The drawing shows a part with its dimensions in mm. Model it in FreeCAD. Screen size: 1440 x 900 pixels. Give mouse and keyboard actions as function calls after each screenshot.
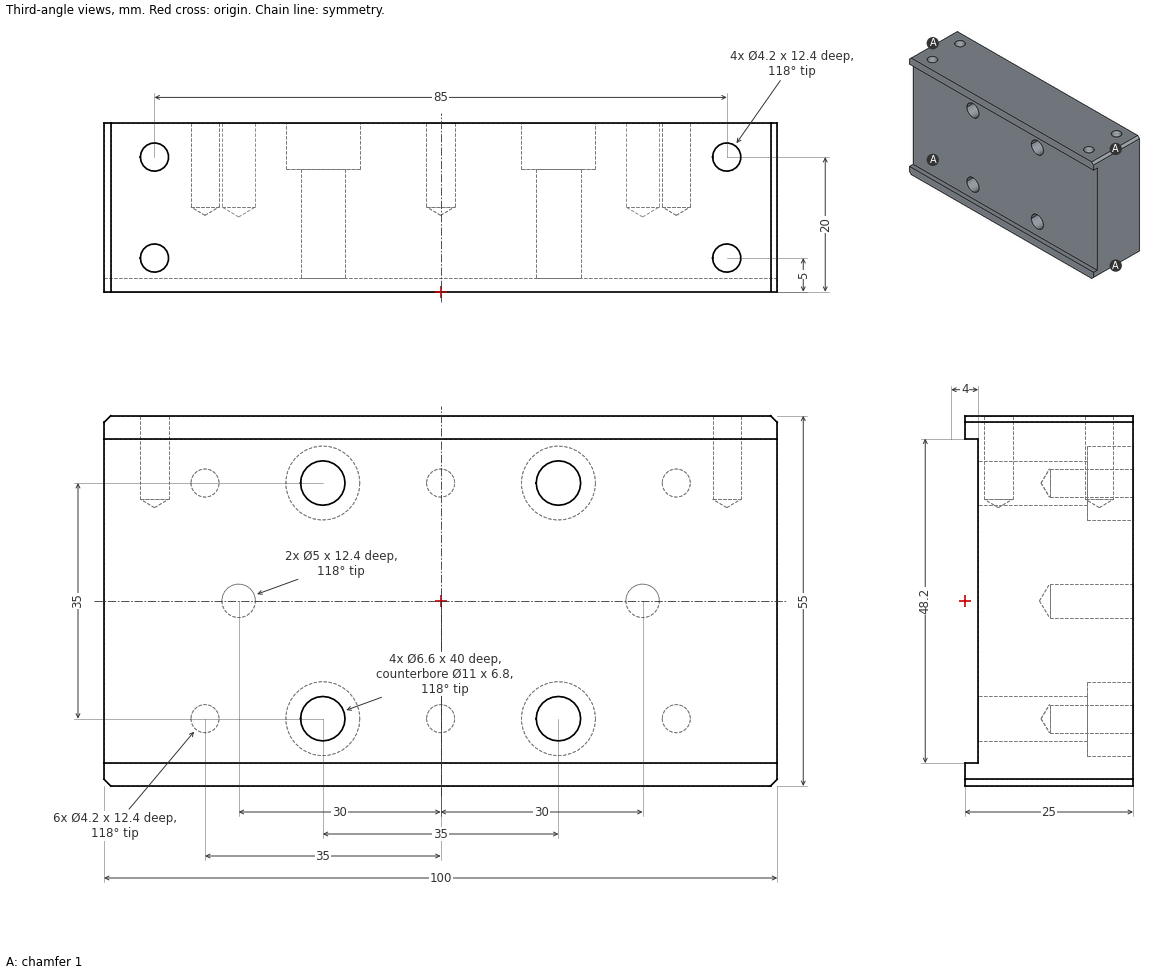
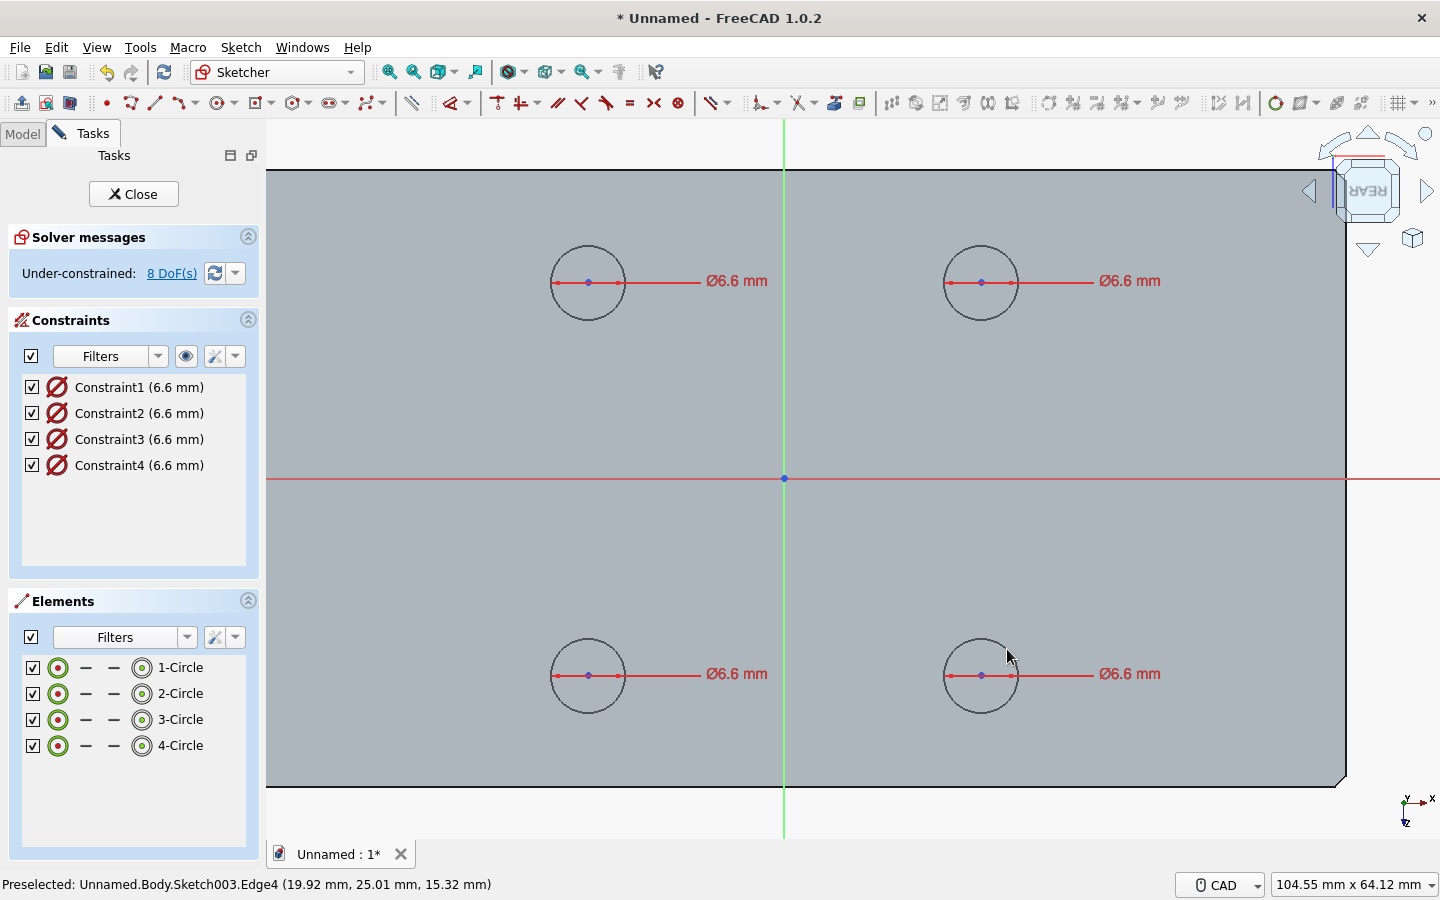
click(588, 283)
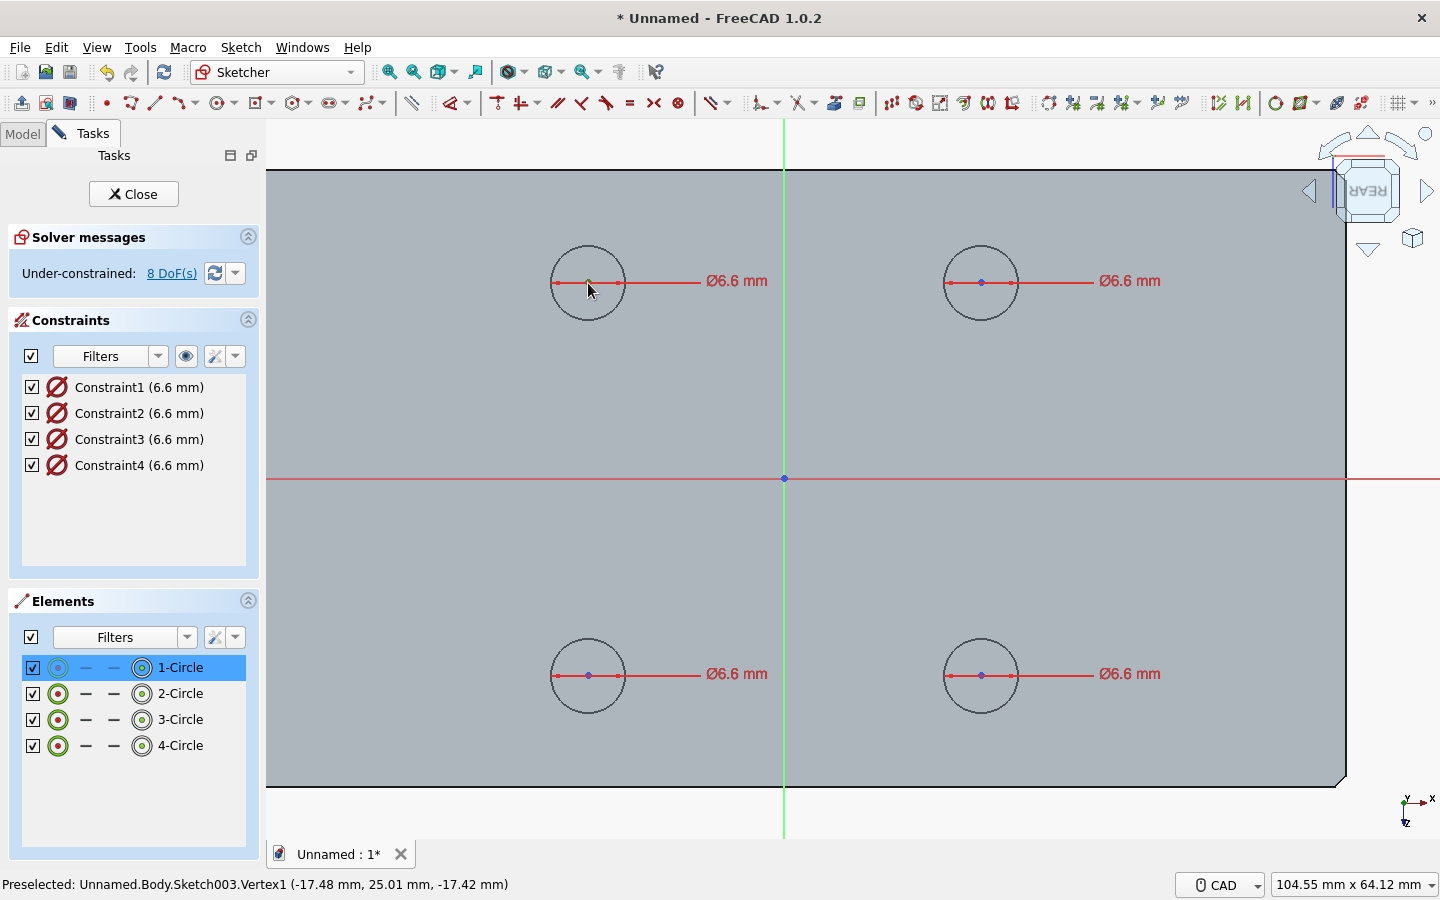
click(981, 283)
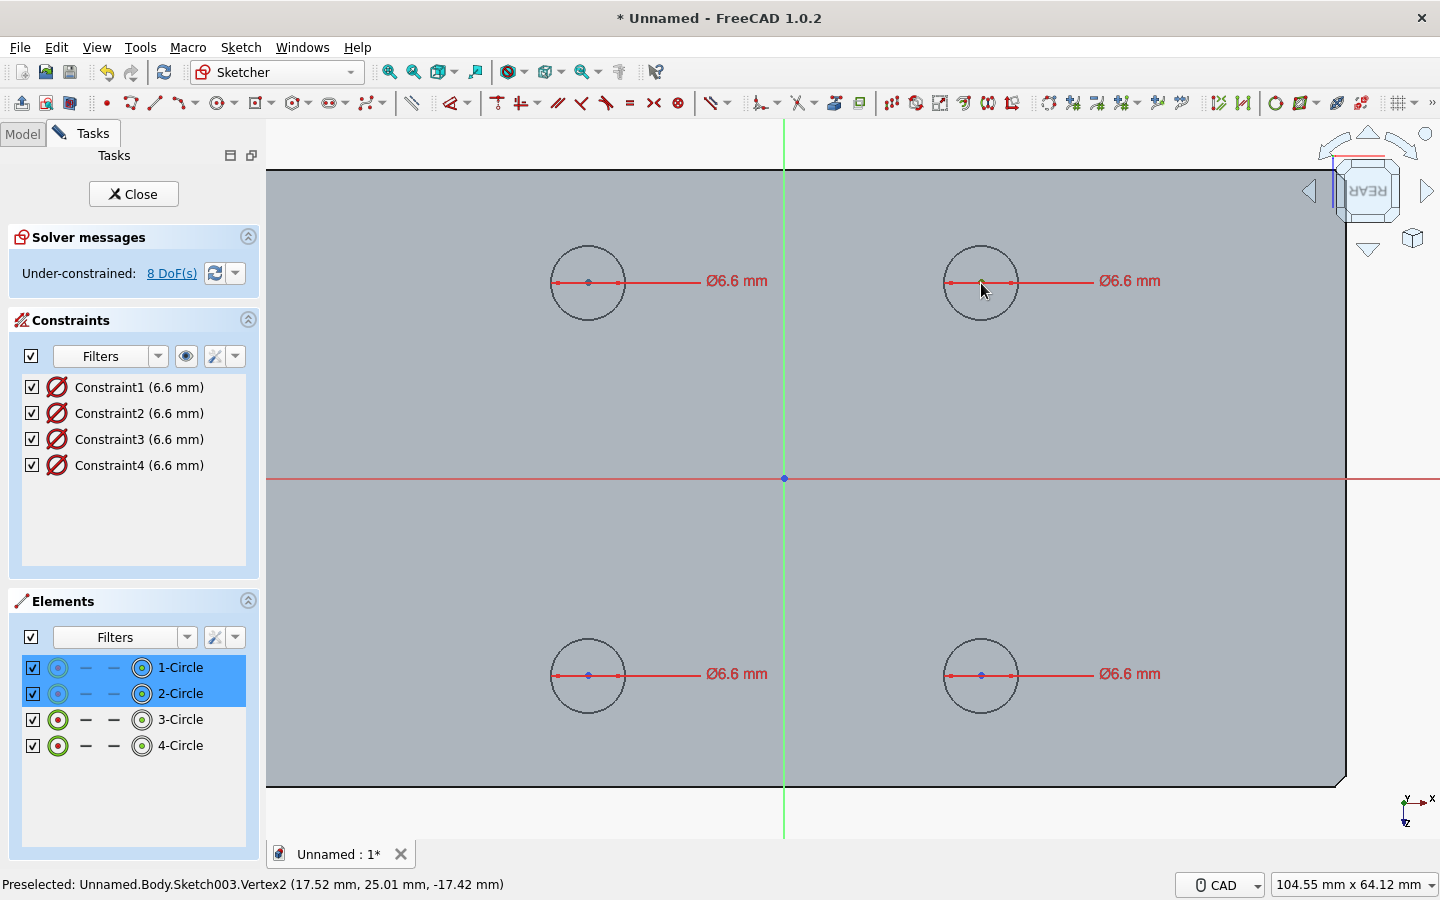
click(784, 764)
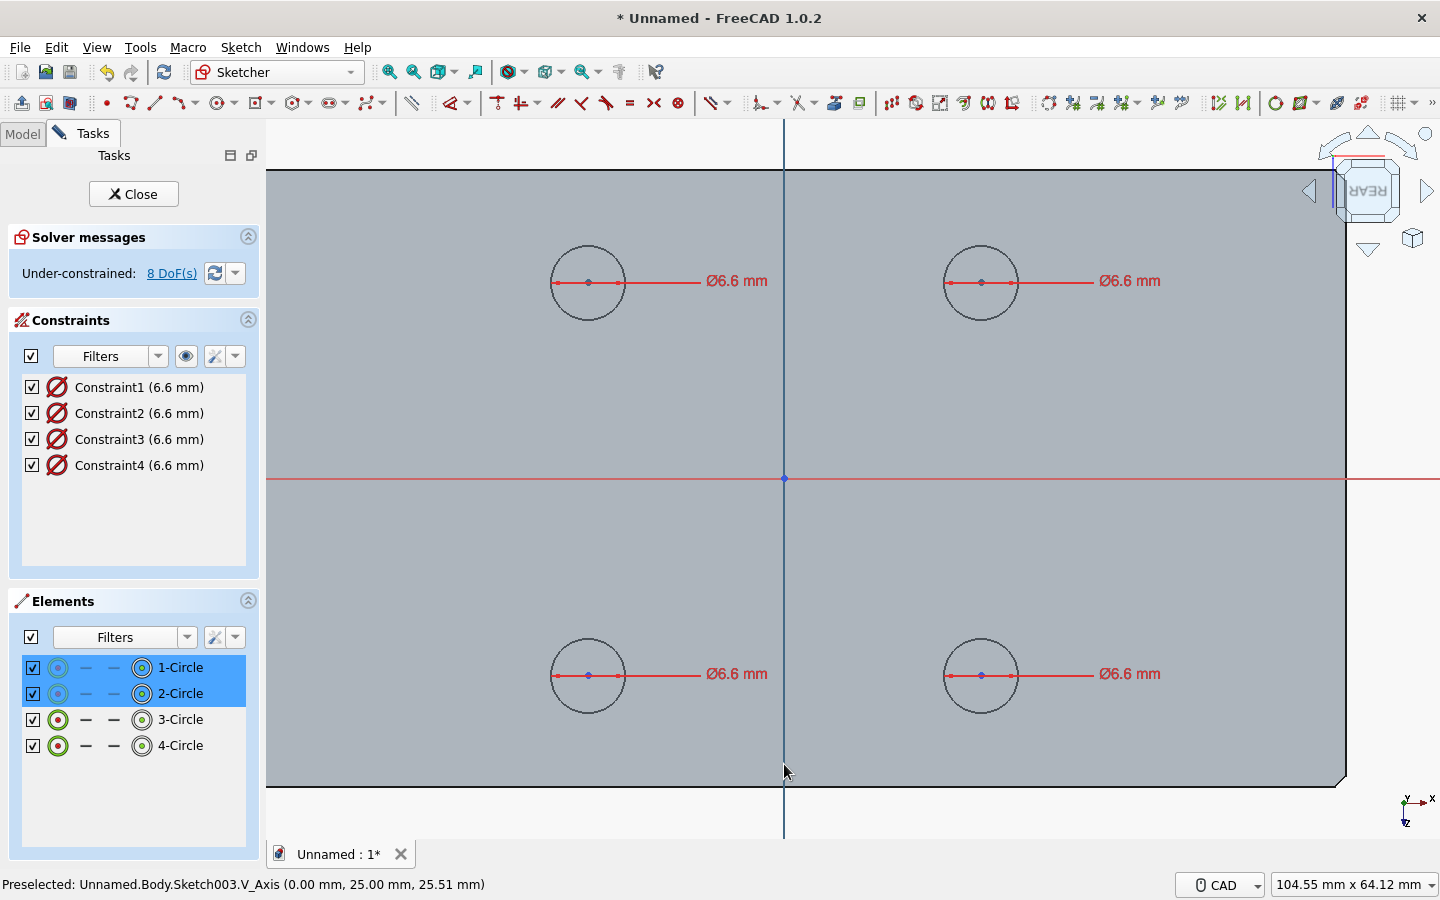
click(654, 104)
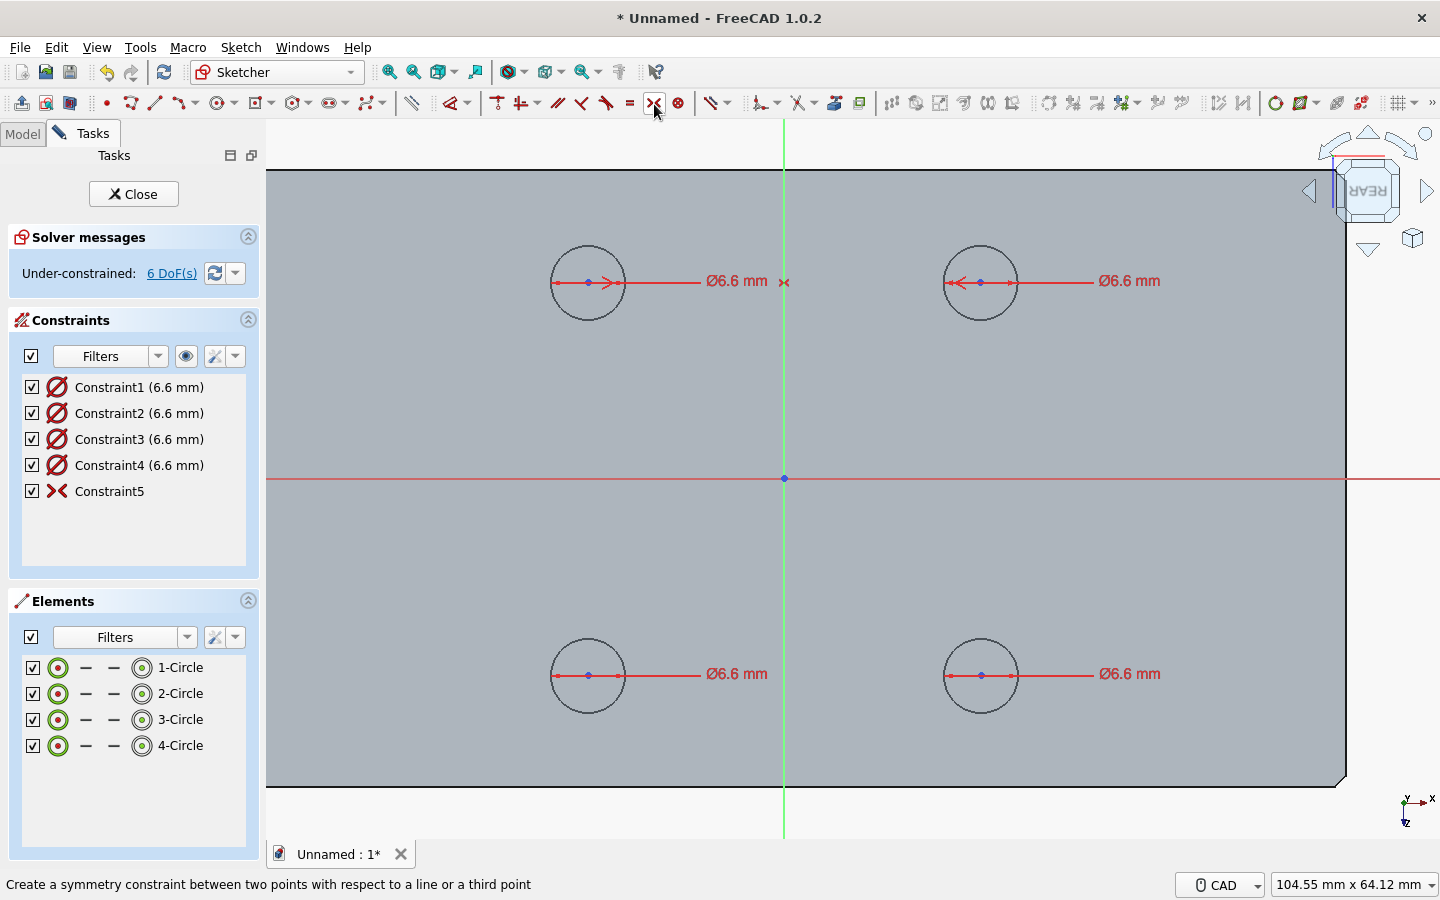
click(588, 283)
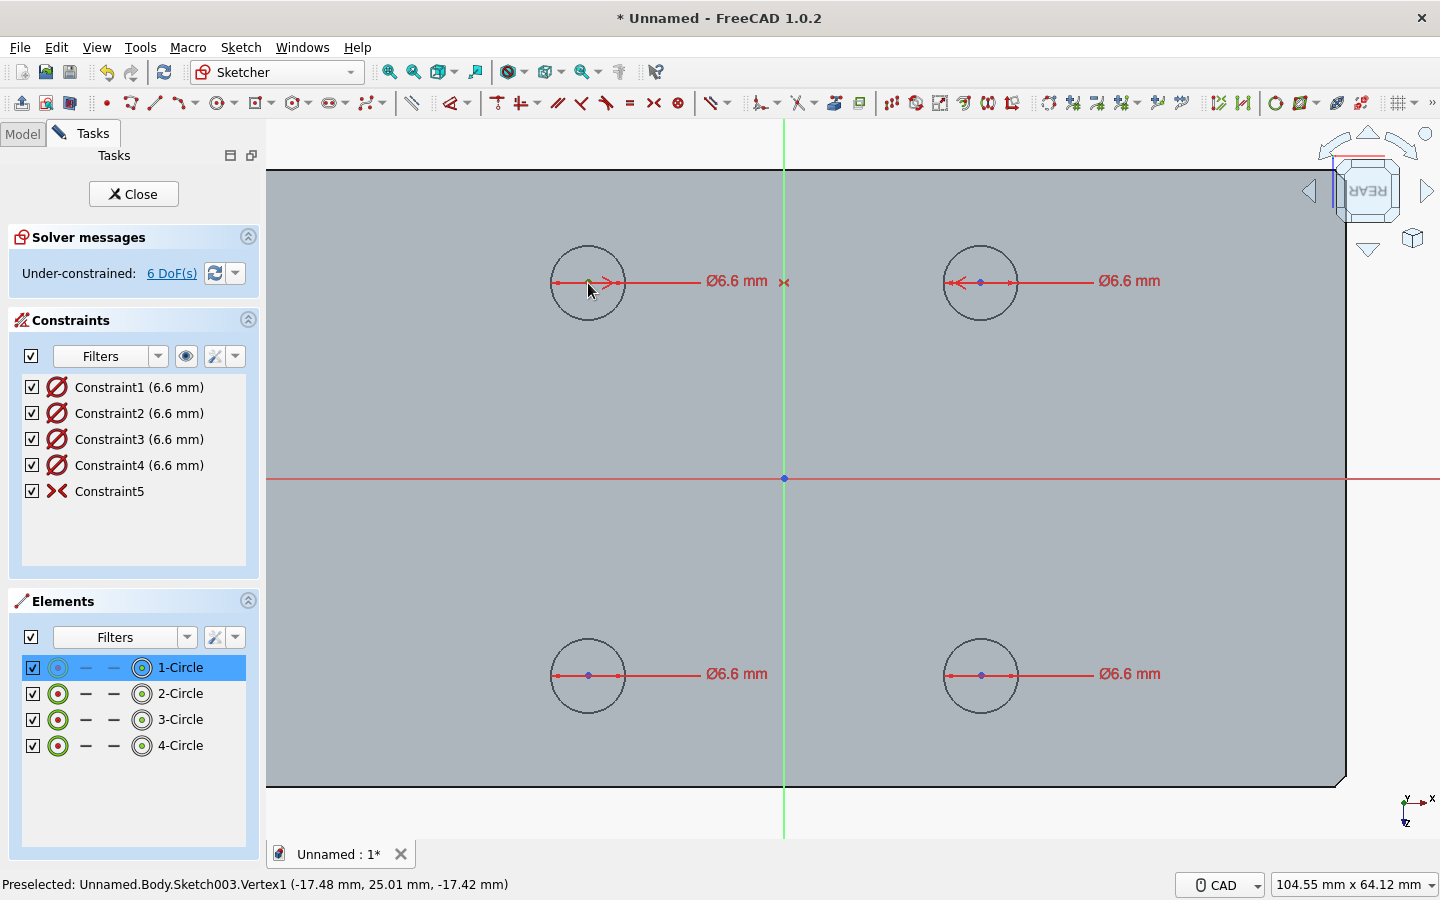
click(588, 676)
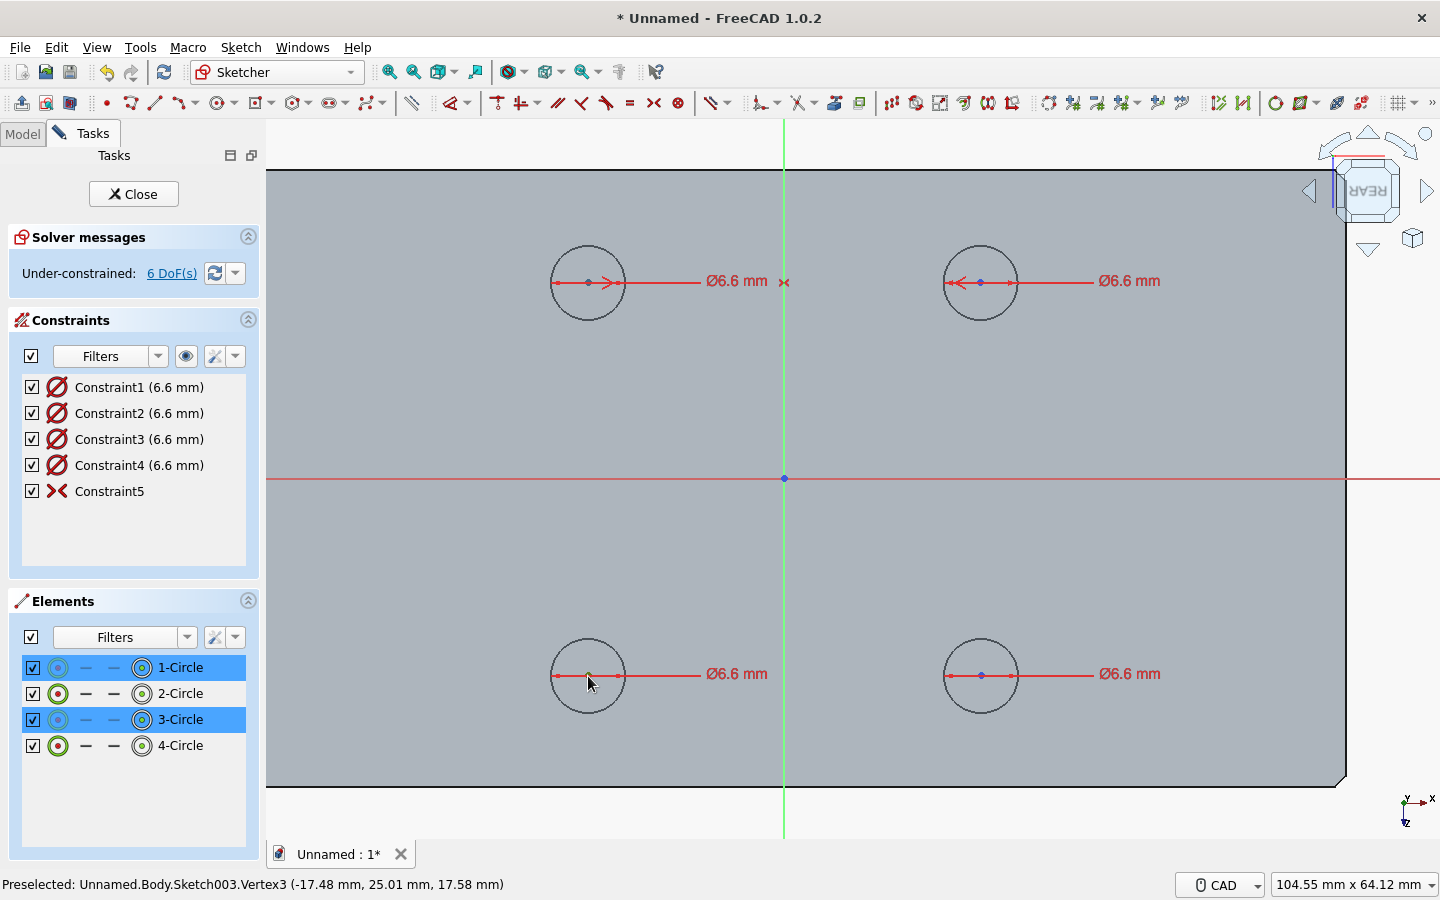
click(364, 479)